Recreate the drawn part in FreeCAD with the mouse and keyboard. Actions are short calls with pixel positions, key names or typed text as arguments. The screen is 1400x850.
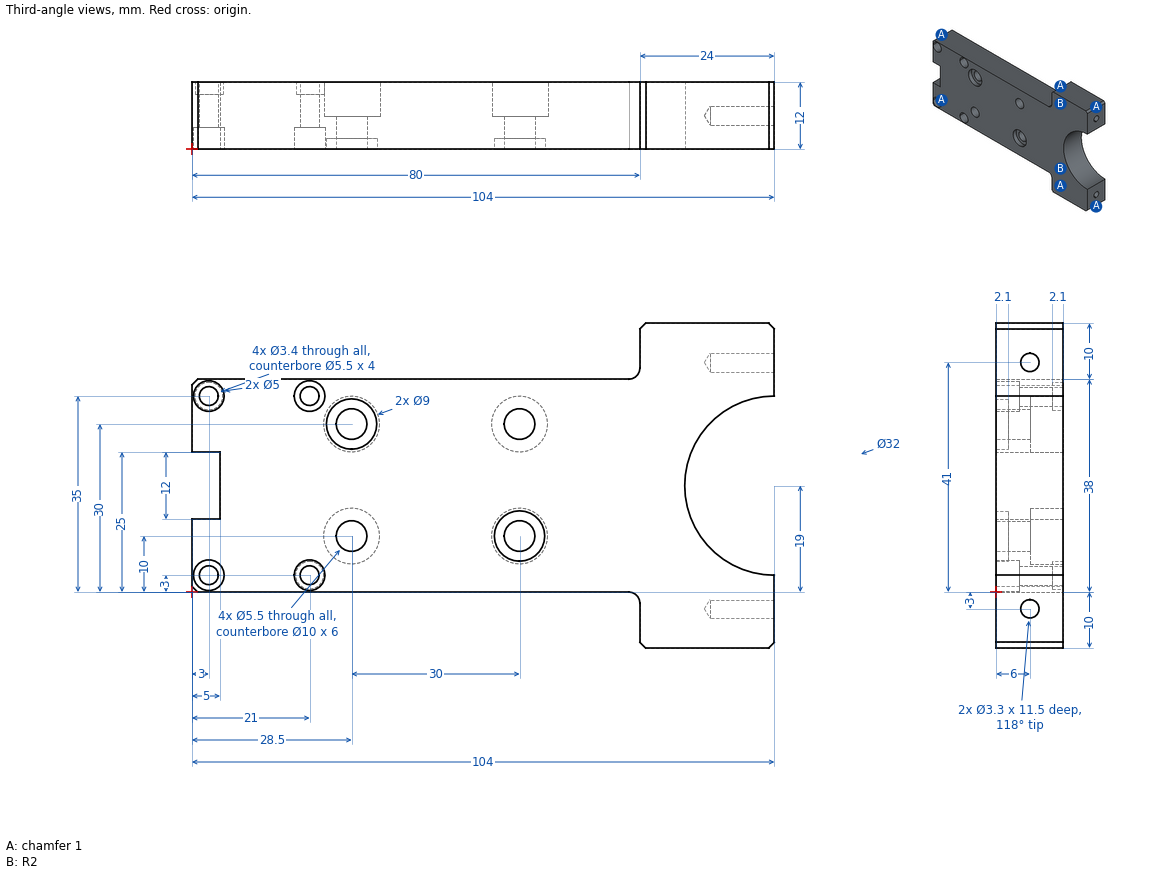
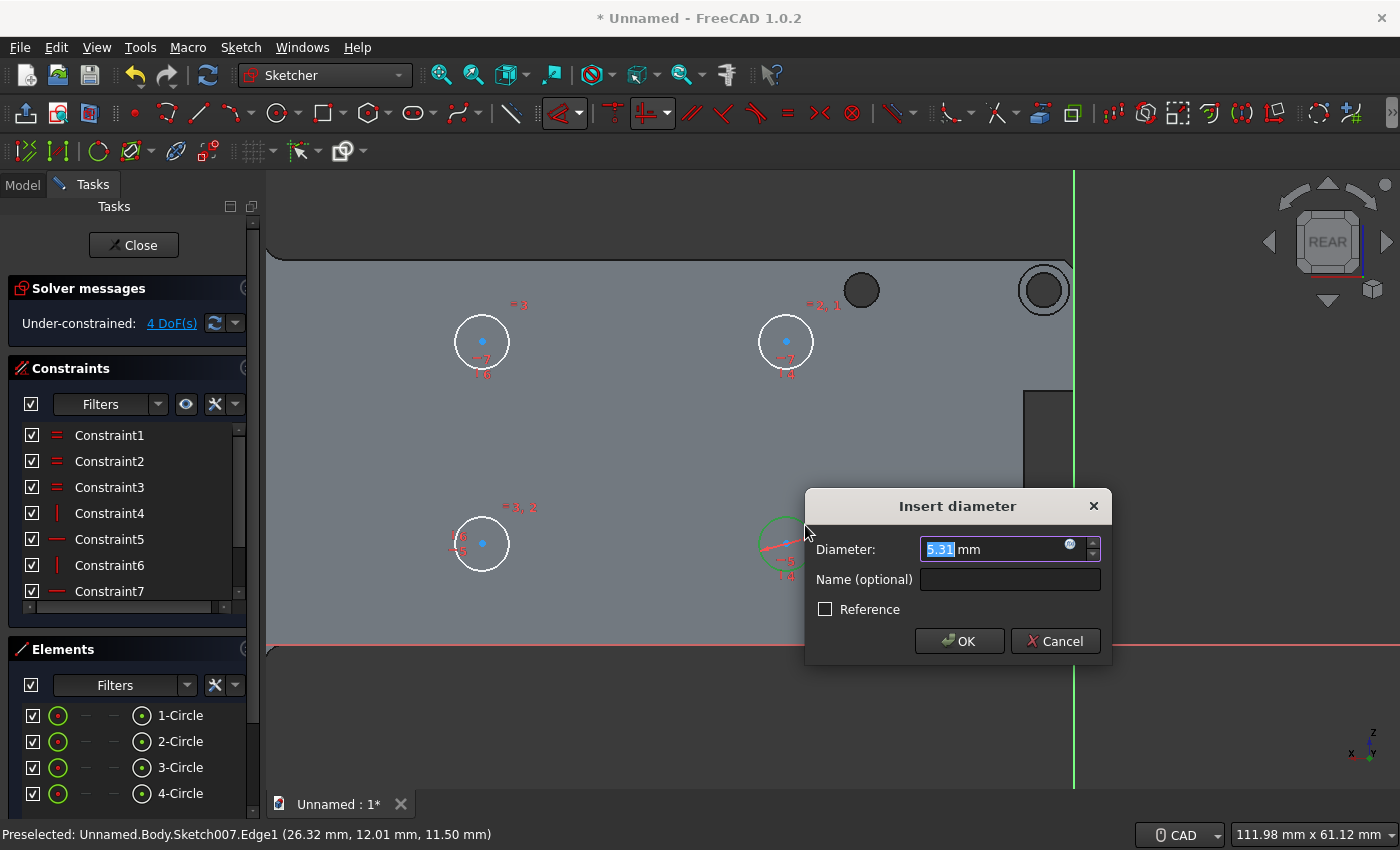
text(5.5)
key(Return)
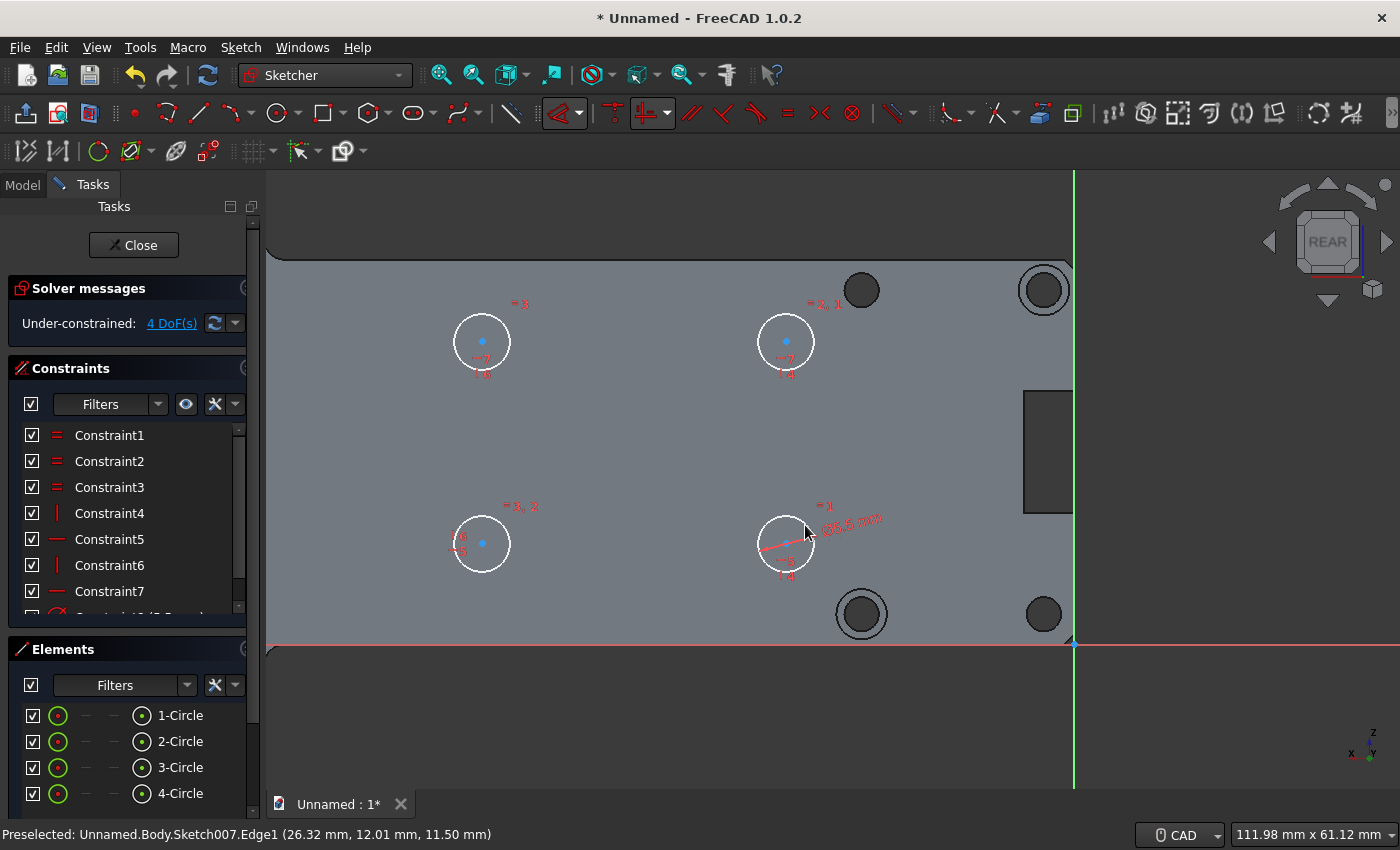
click(786, 544)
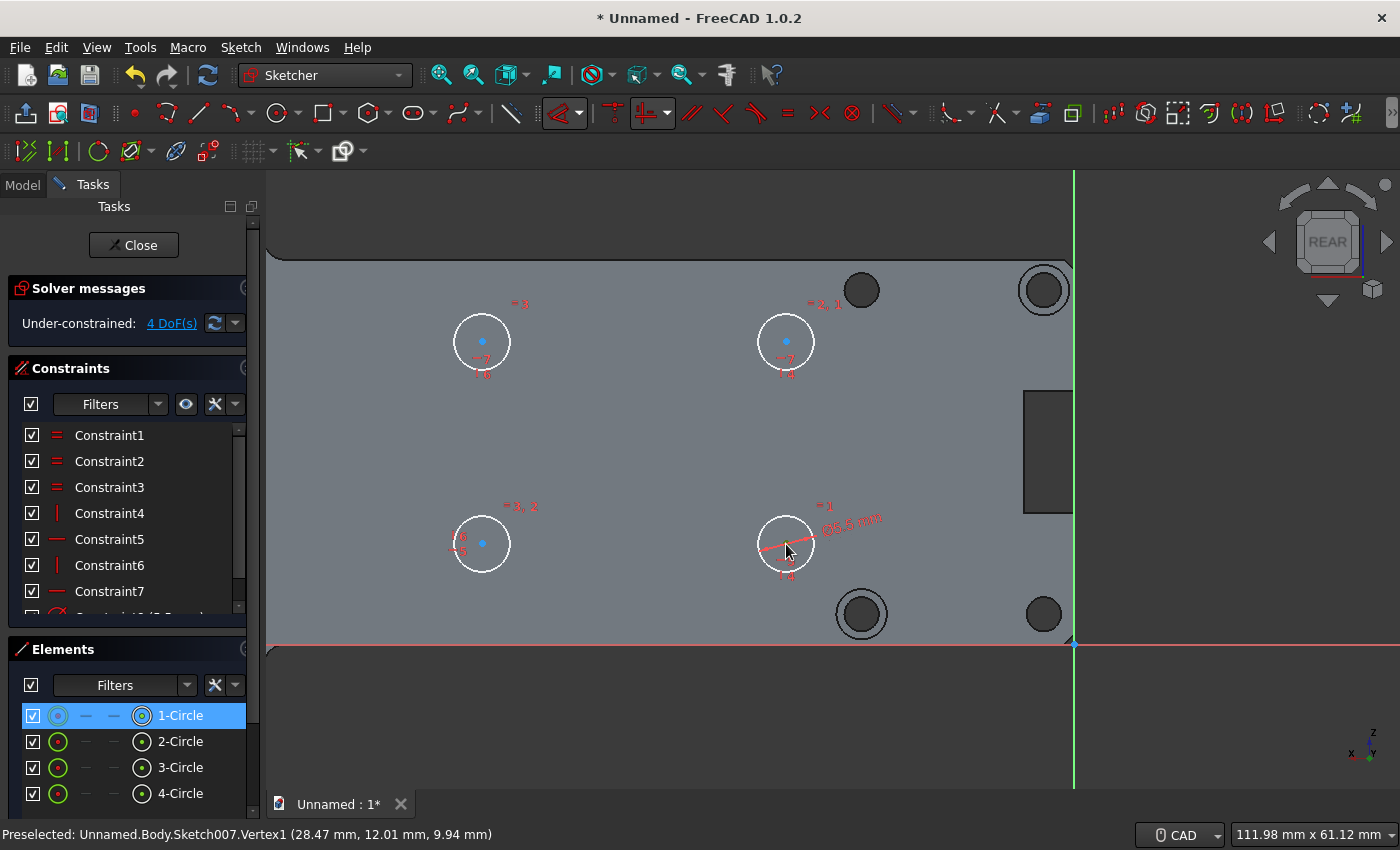
click(582, 114)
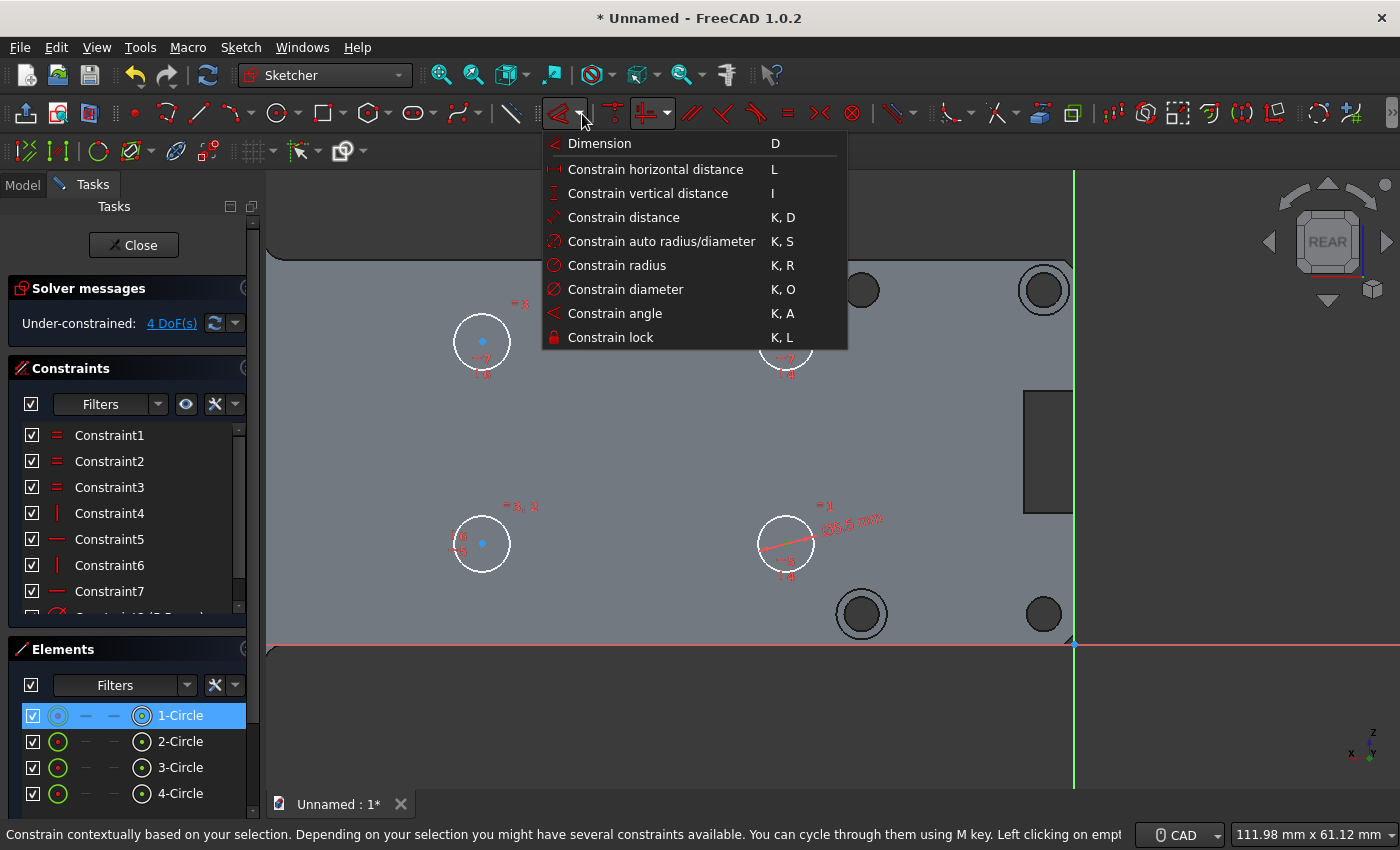
click(695, 193)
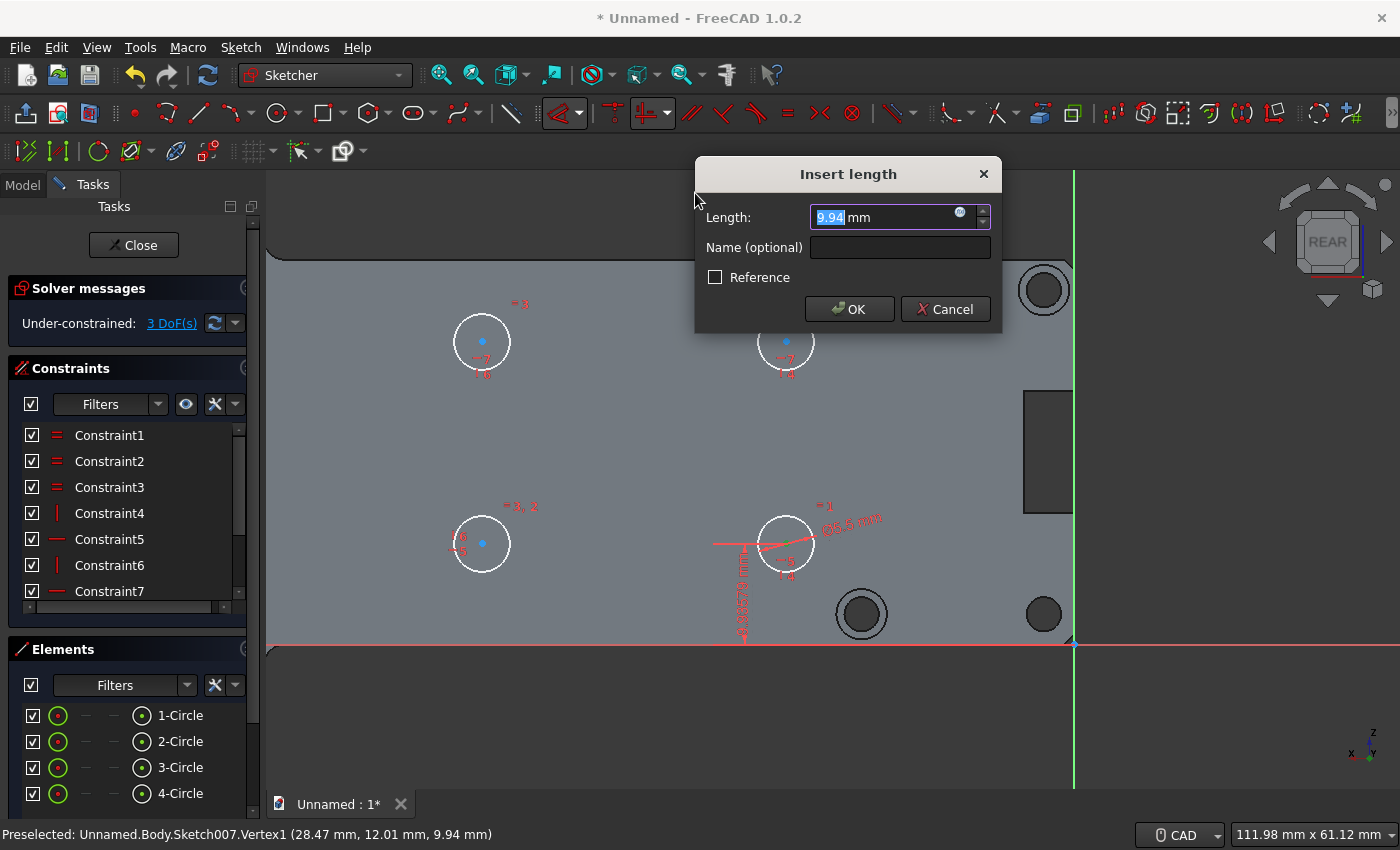
text(10)
key(Return)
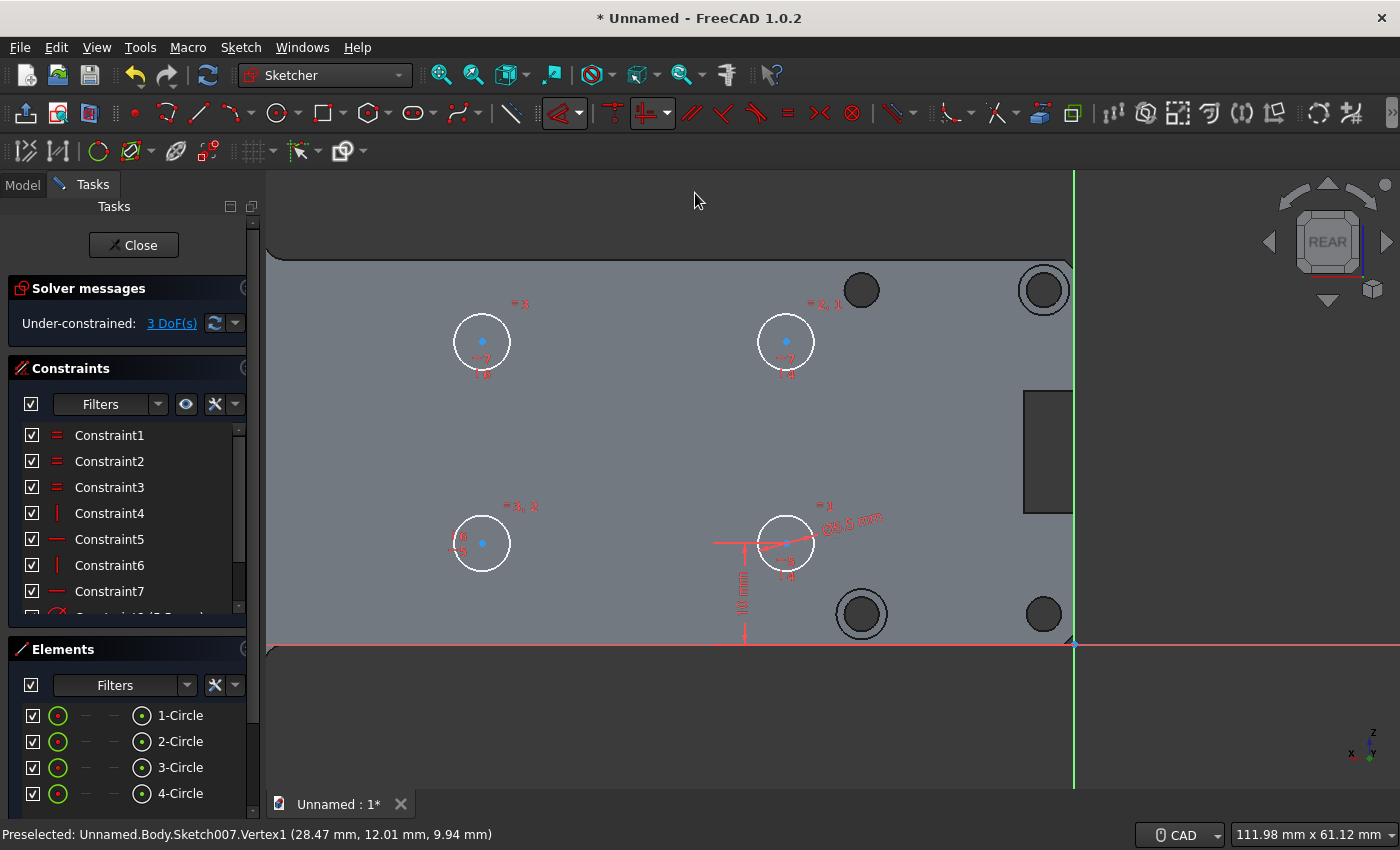
click(786, 342)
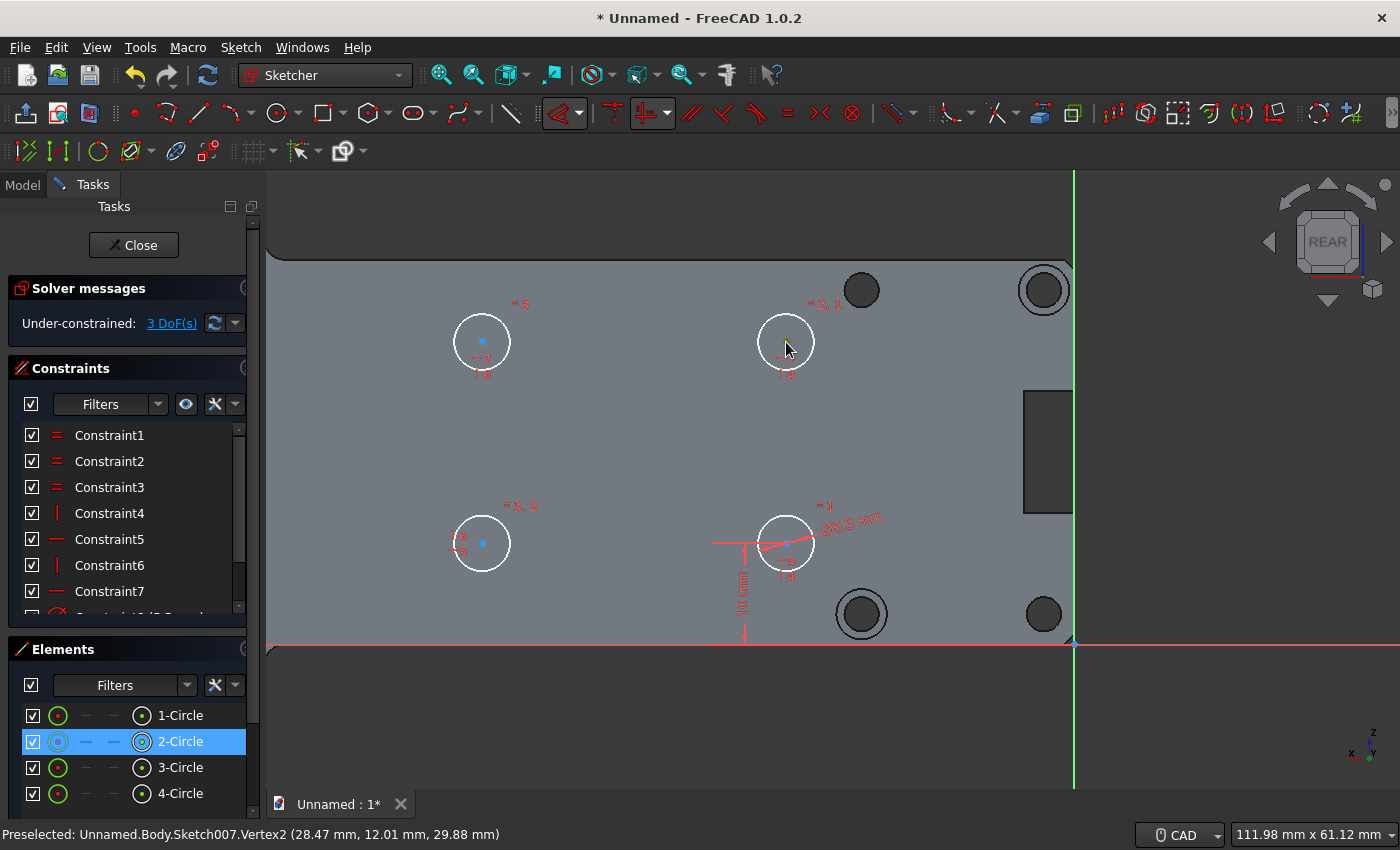
key(i)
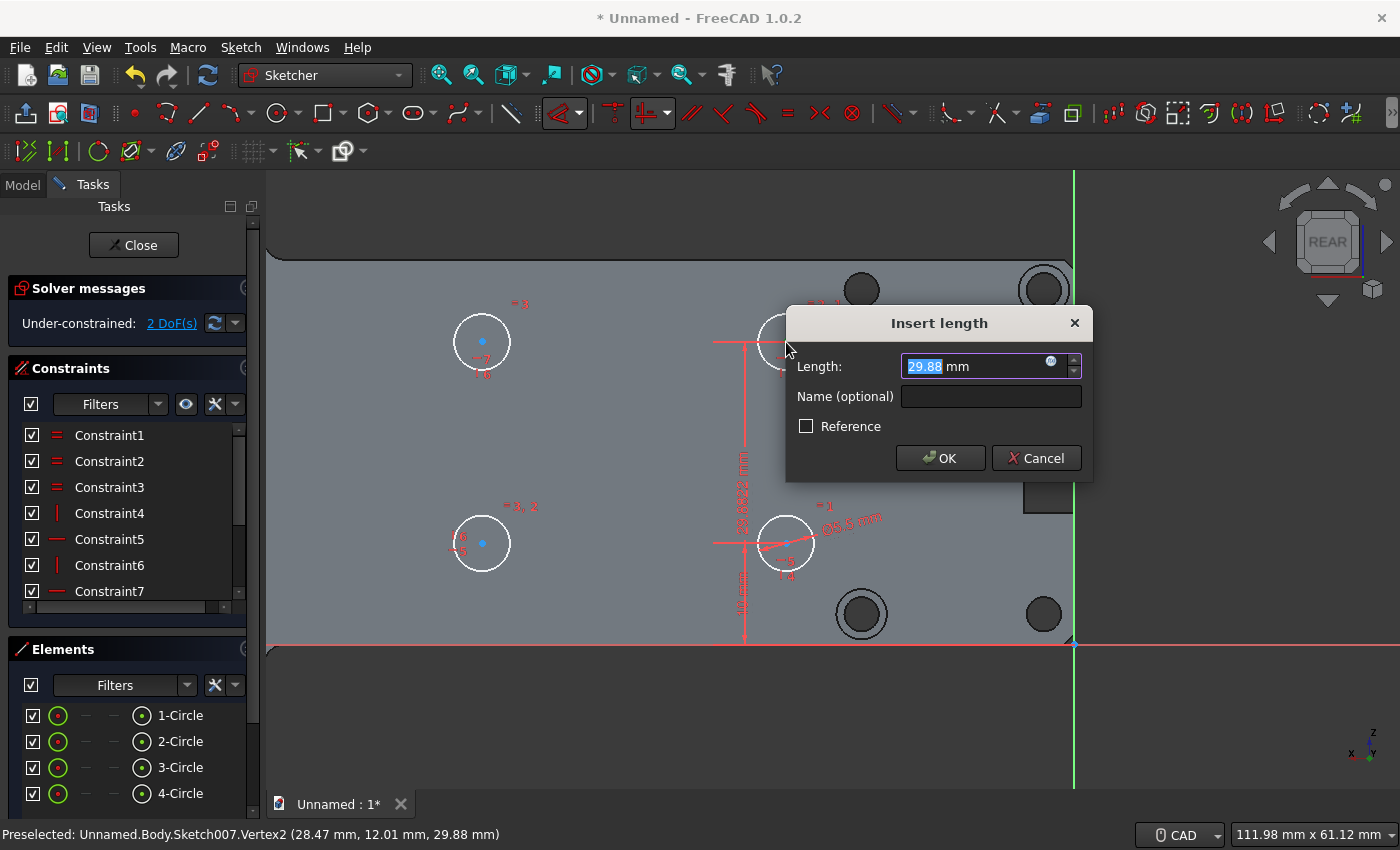
text(30)
key(Return)